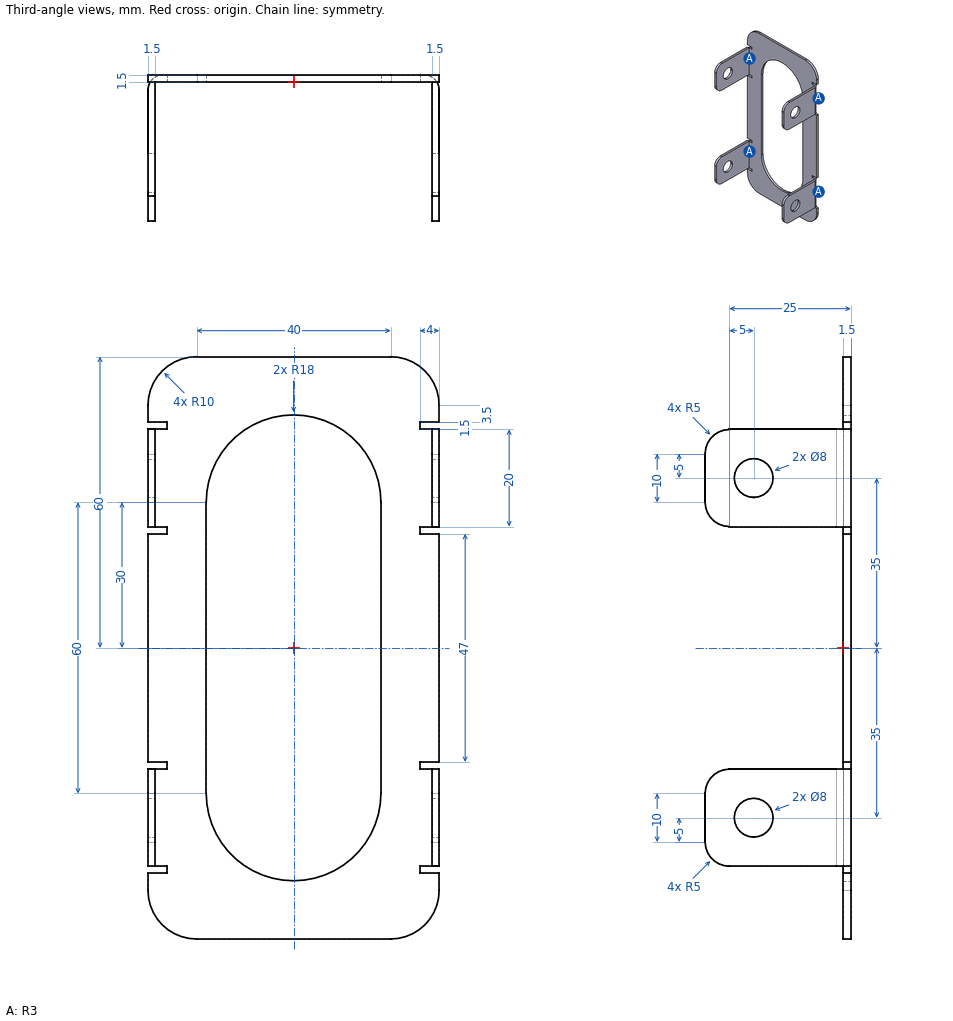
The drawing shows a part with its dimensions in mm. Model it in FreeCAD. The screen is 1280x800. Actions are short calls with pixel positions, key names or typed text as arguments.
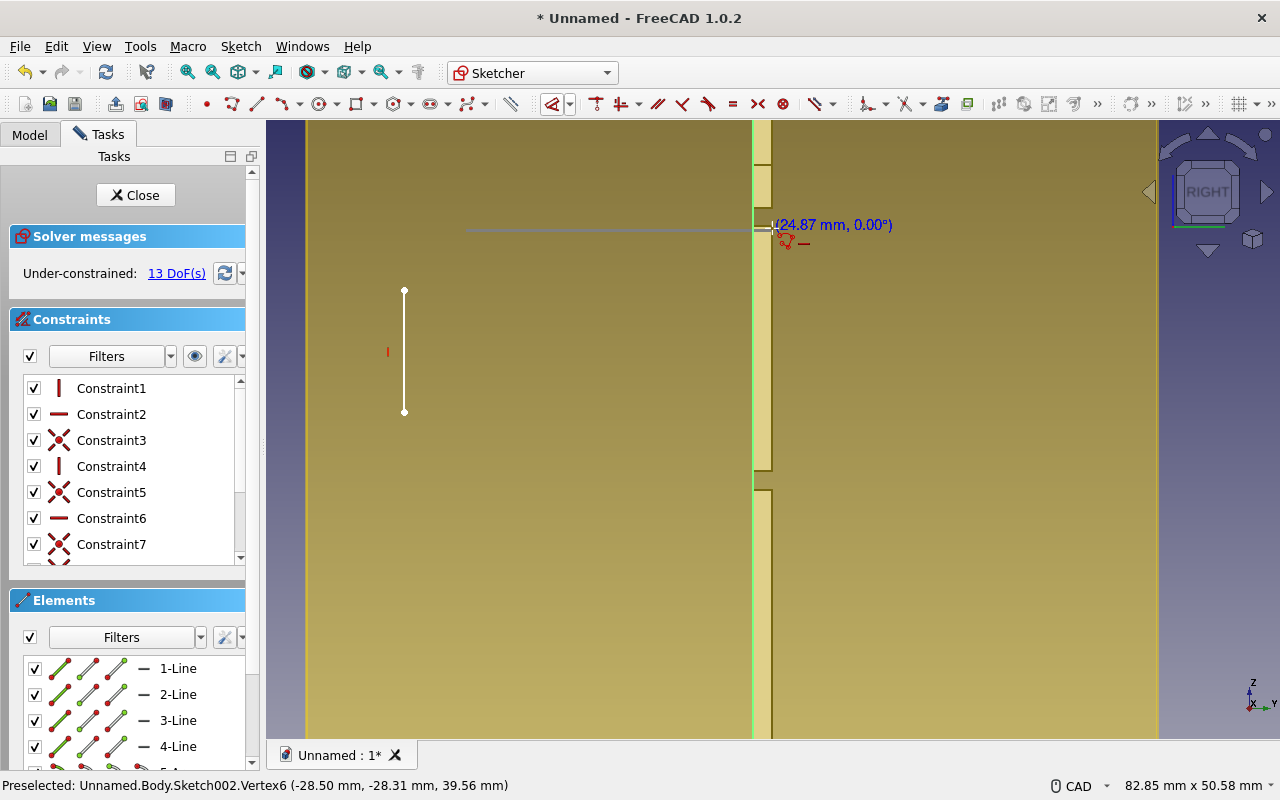
click(772, 228)
click(772, 471)
click(466, 471)
right_click(466, 471)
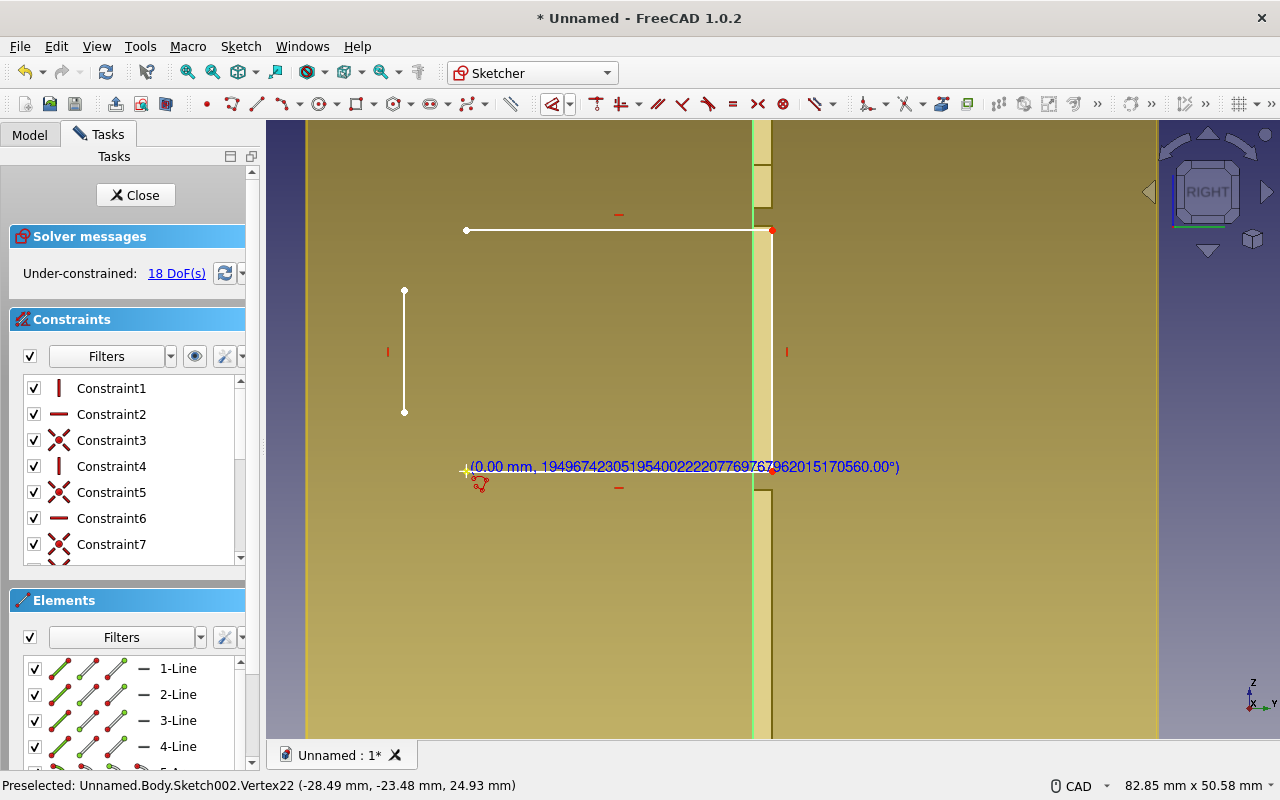
click(282, 104)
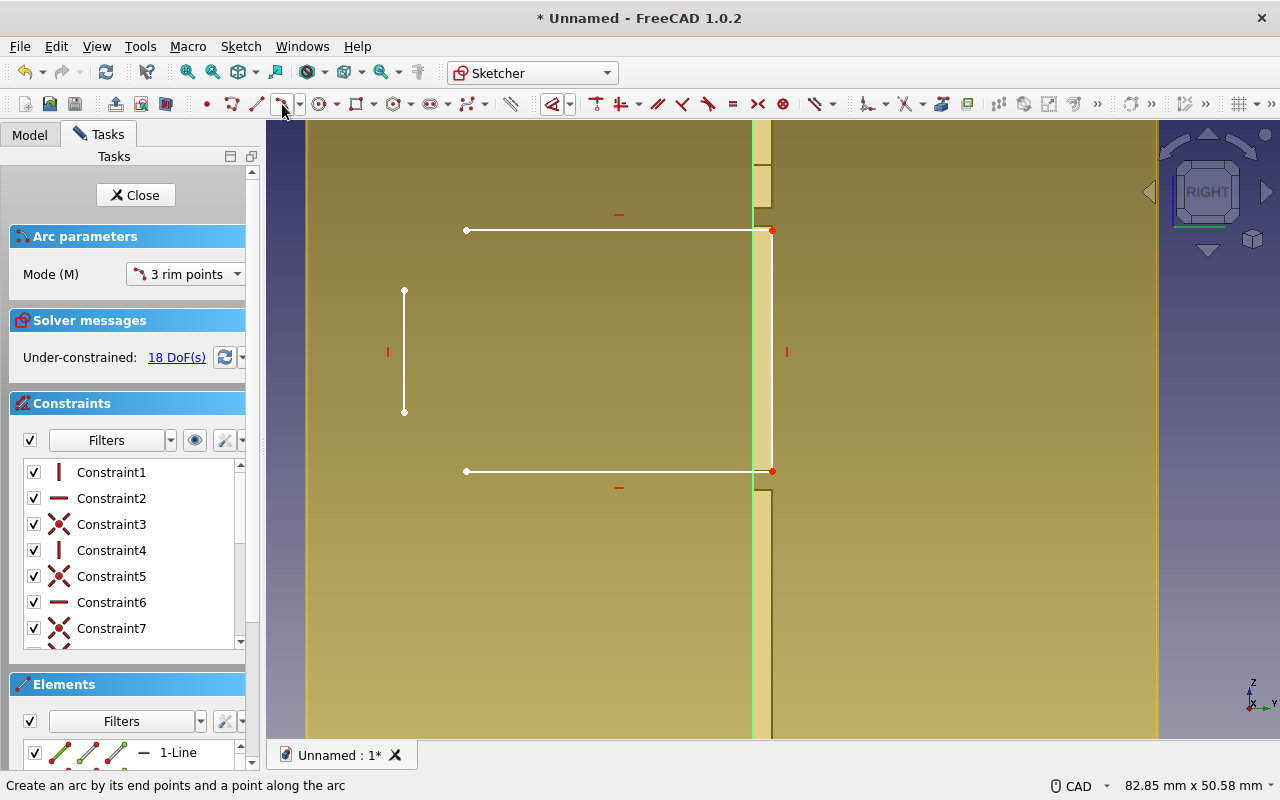
click(404, 290)
click(467, 230)
click(422, 244)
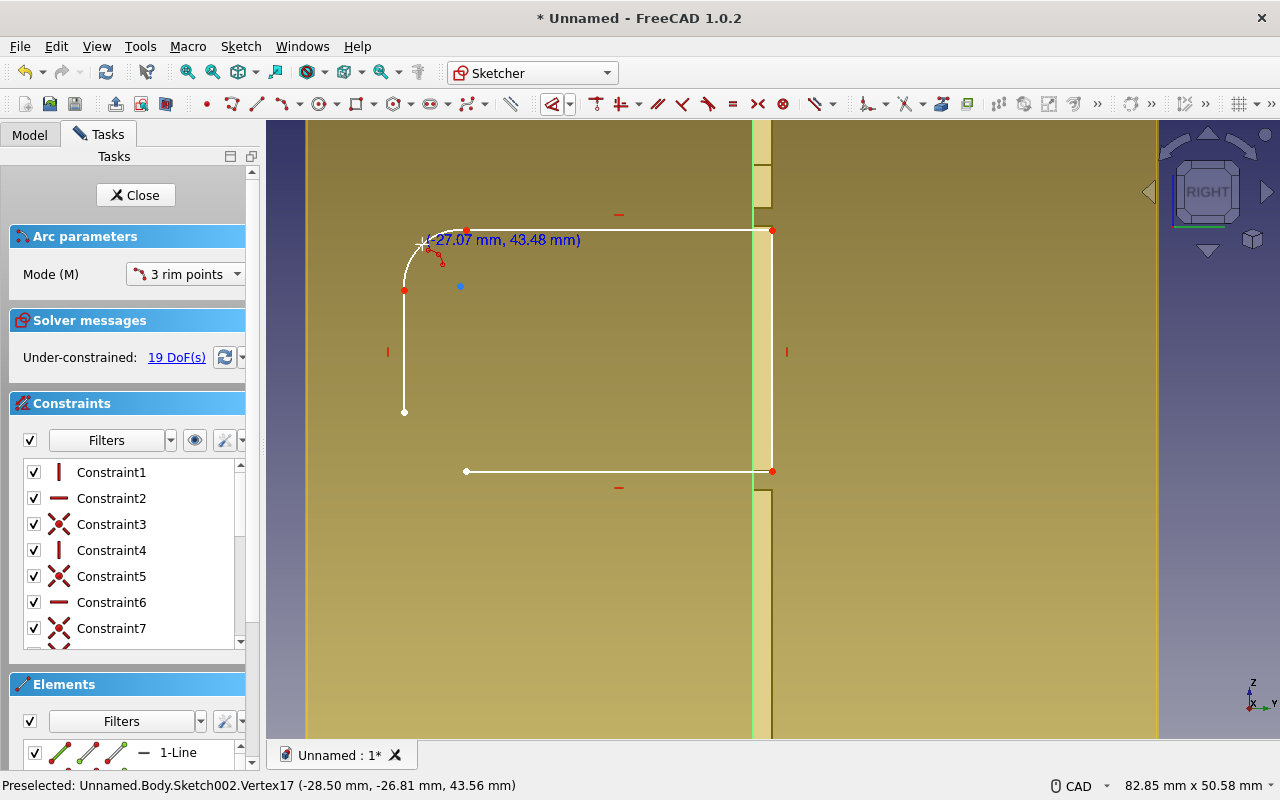
click(466, 472)
click(404, 413)
click(422, 453)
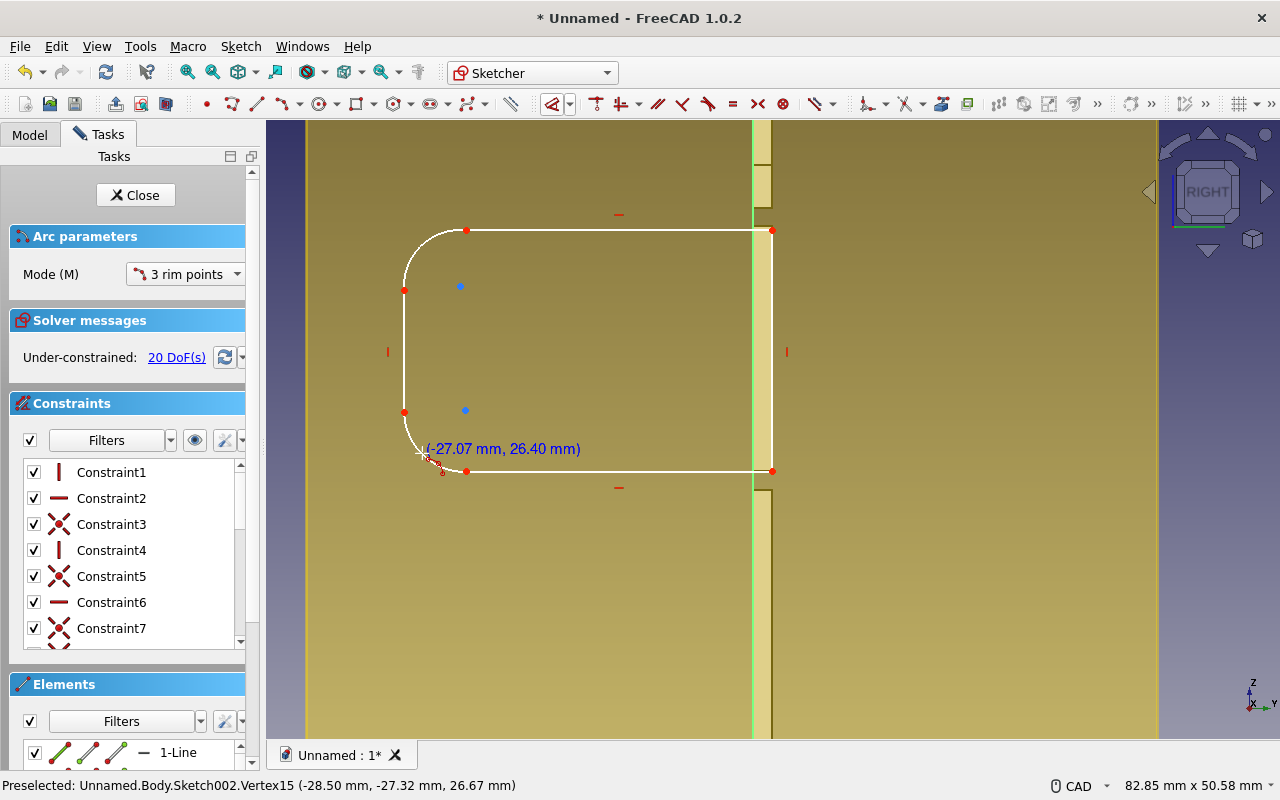
key(g)
key(c)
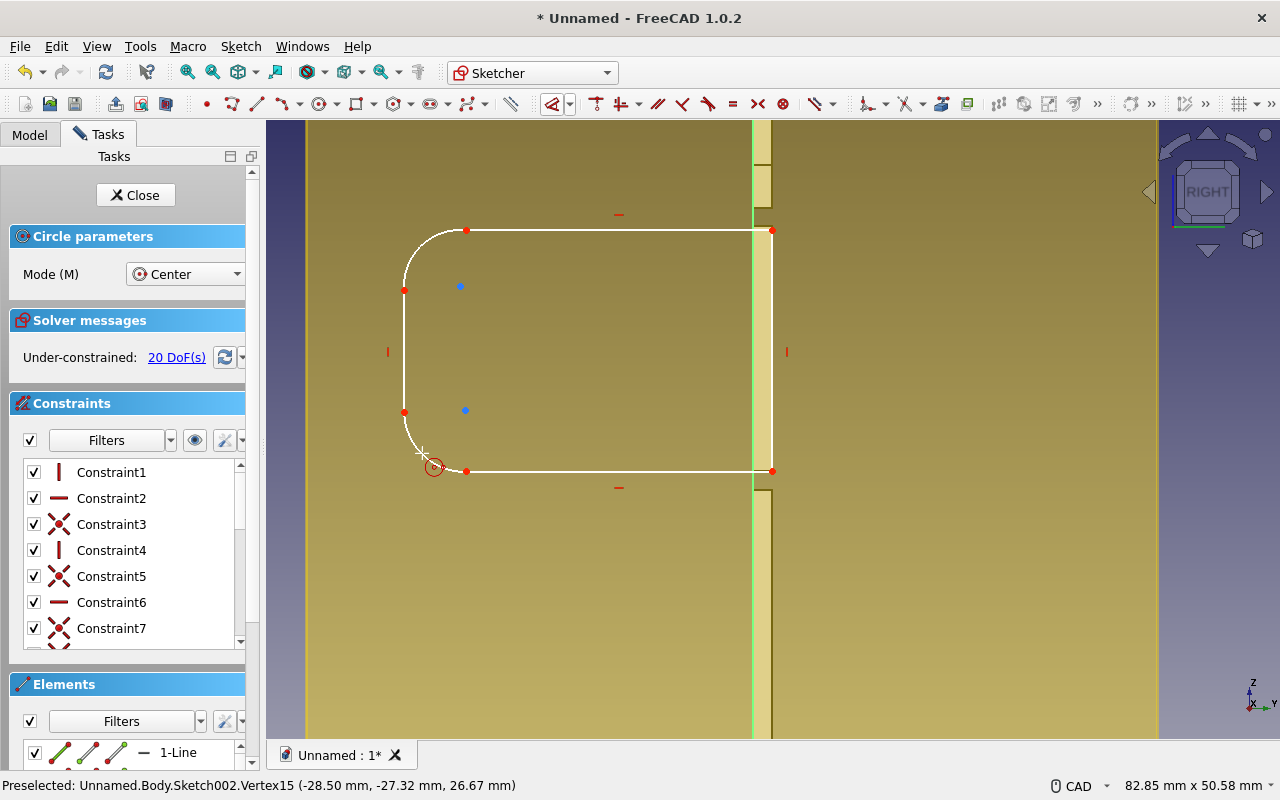
scroll(772, 227, down, 5)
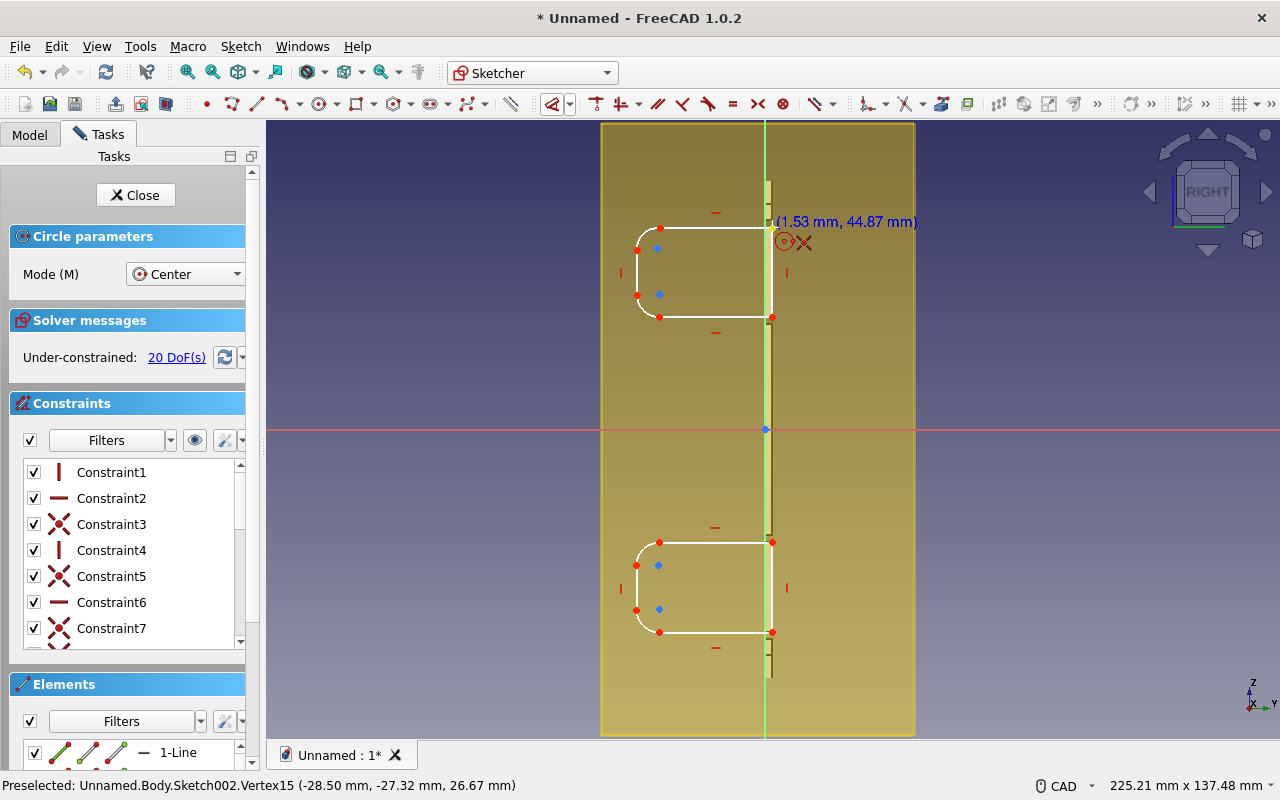
scroll(682, 587, up, 2)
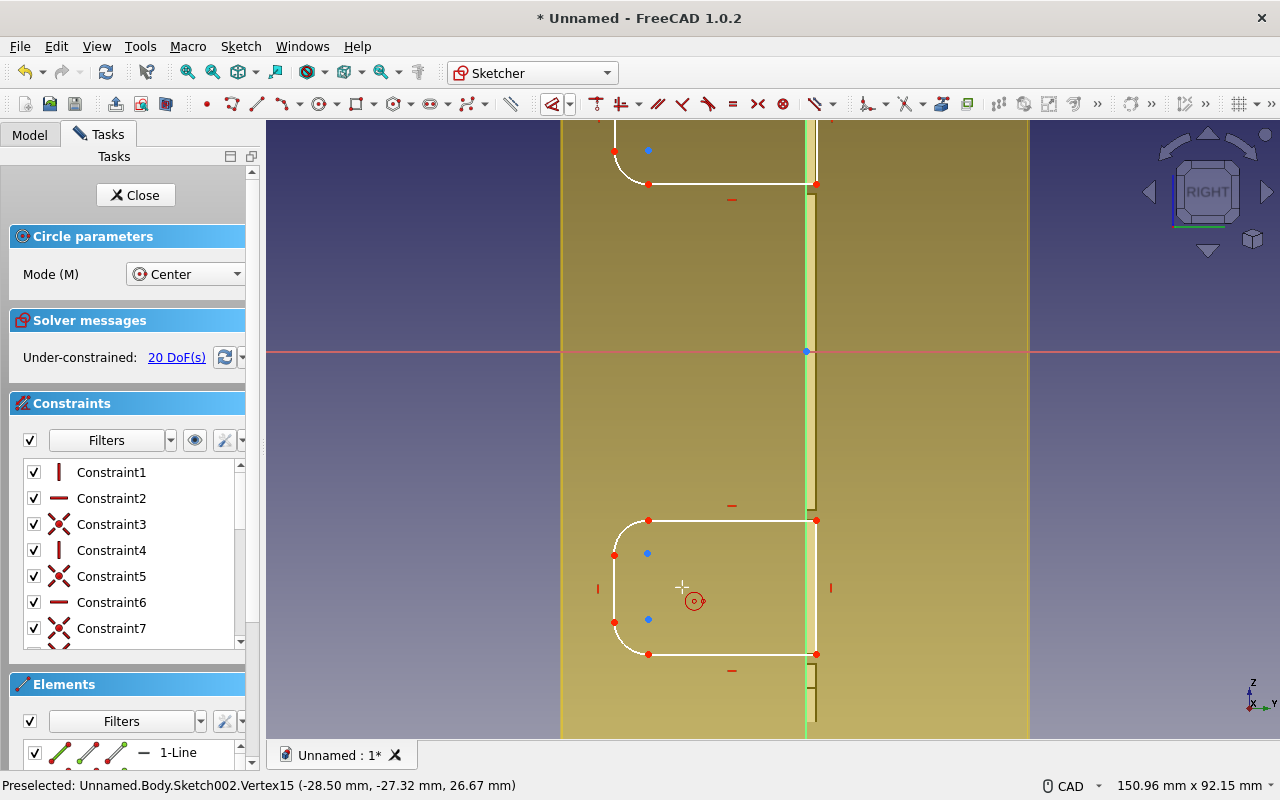
click(682, 587)
move(701, 568)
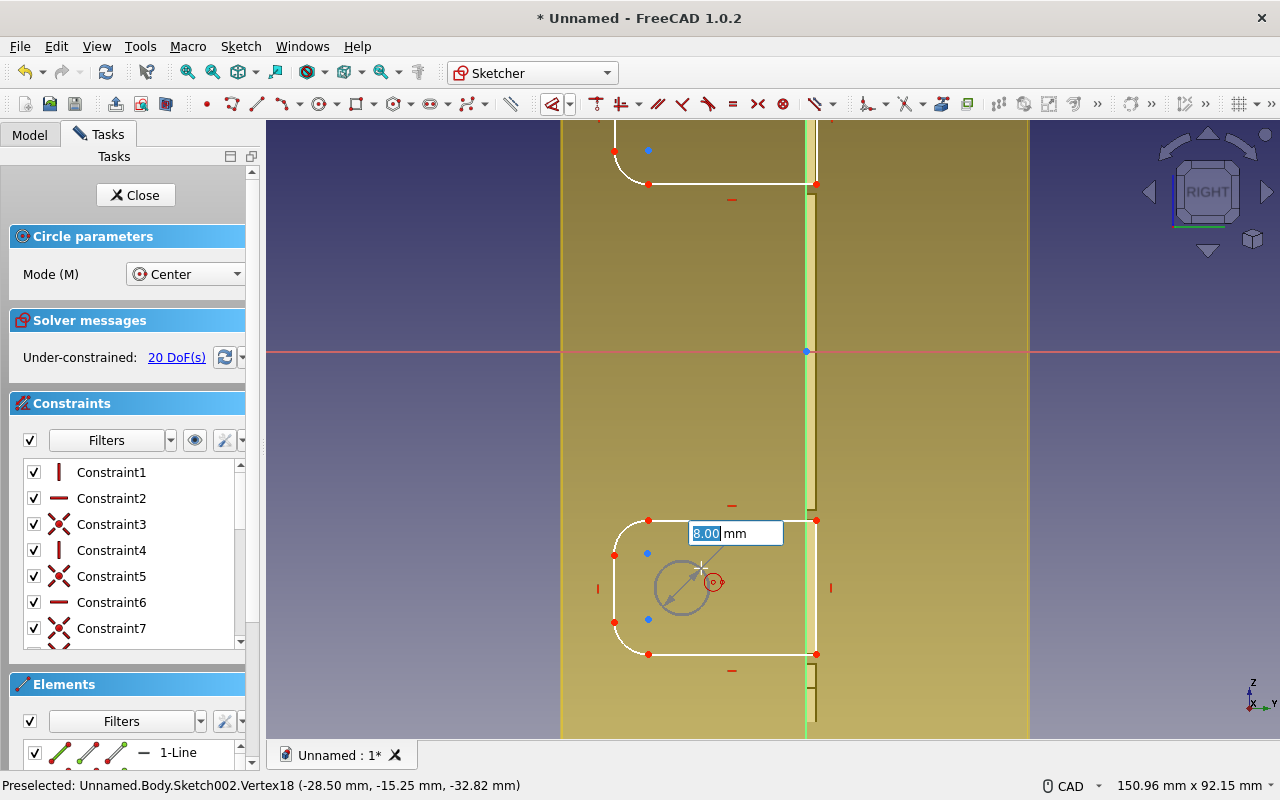
text(8)
key(Return)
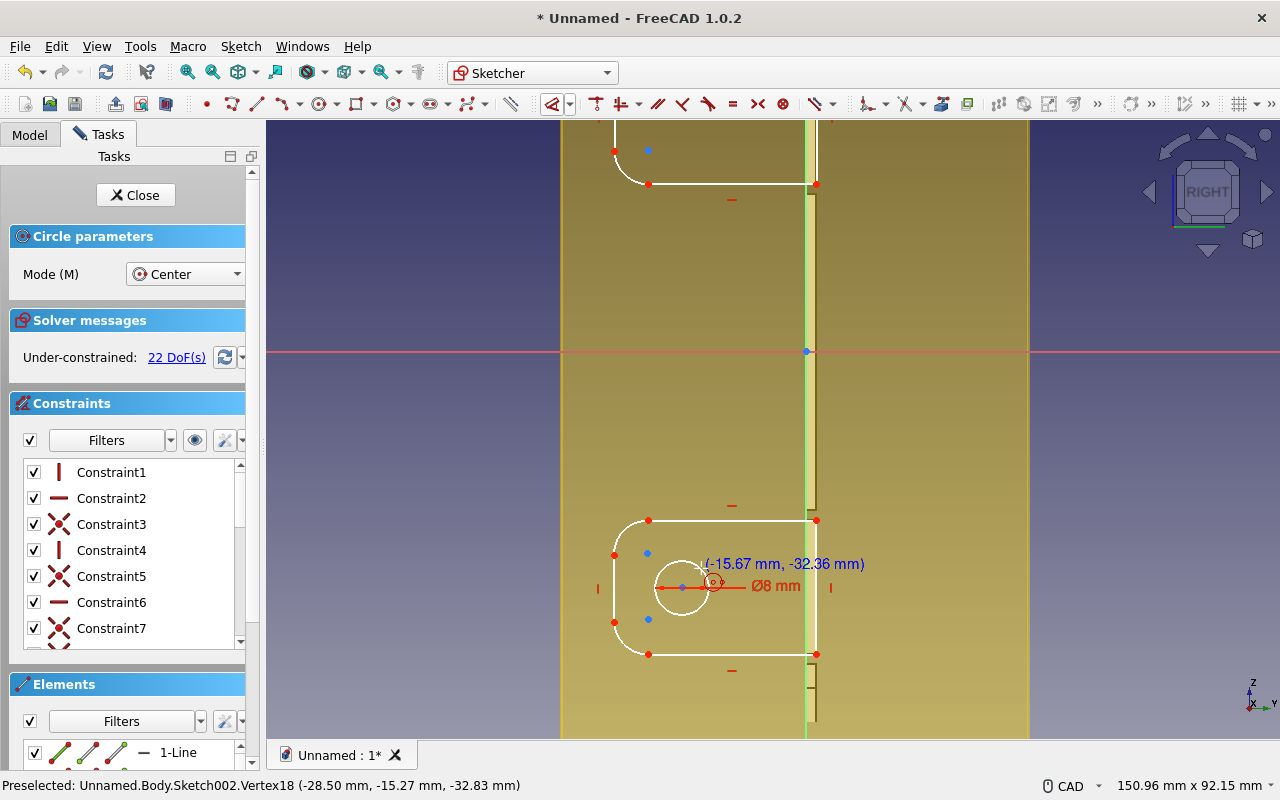
scroll(682, 588, down, 2)